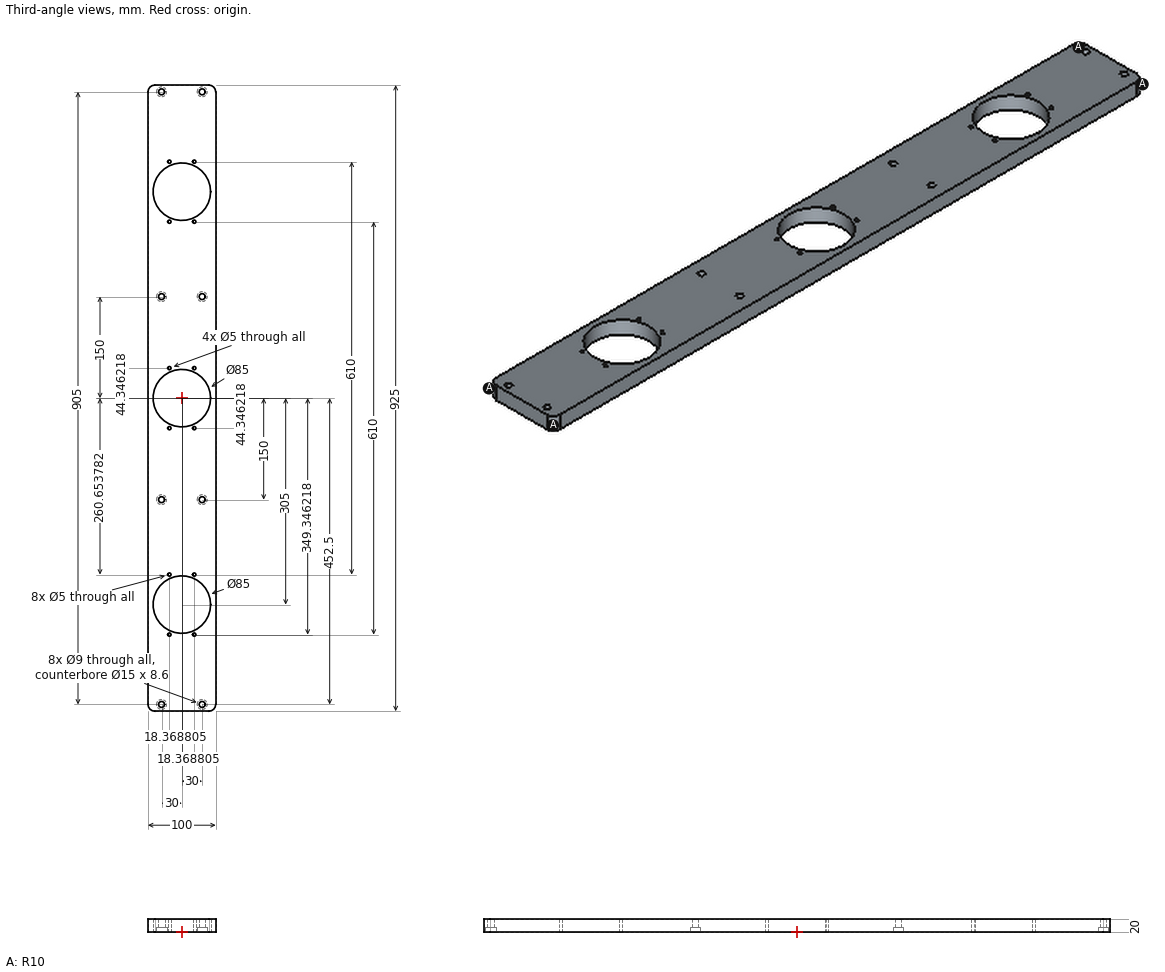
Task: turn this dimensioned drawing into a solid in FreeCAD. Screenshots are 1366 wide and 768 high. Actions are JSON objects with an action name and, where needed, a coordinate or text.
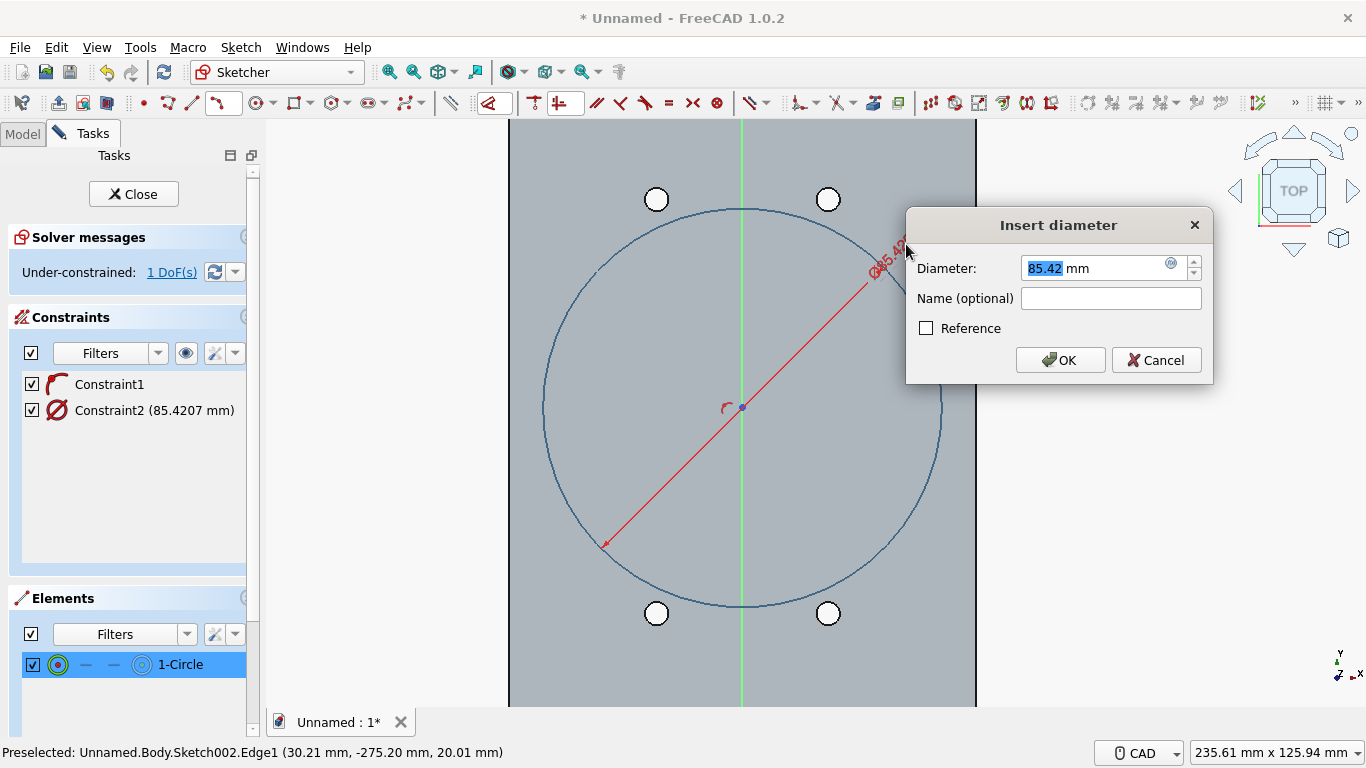
{"action": "type", "text": "85"}
{"action": "key", "text": "Return"}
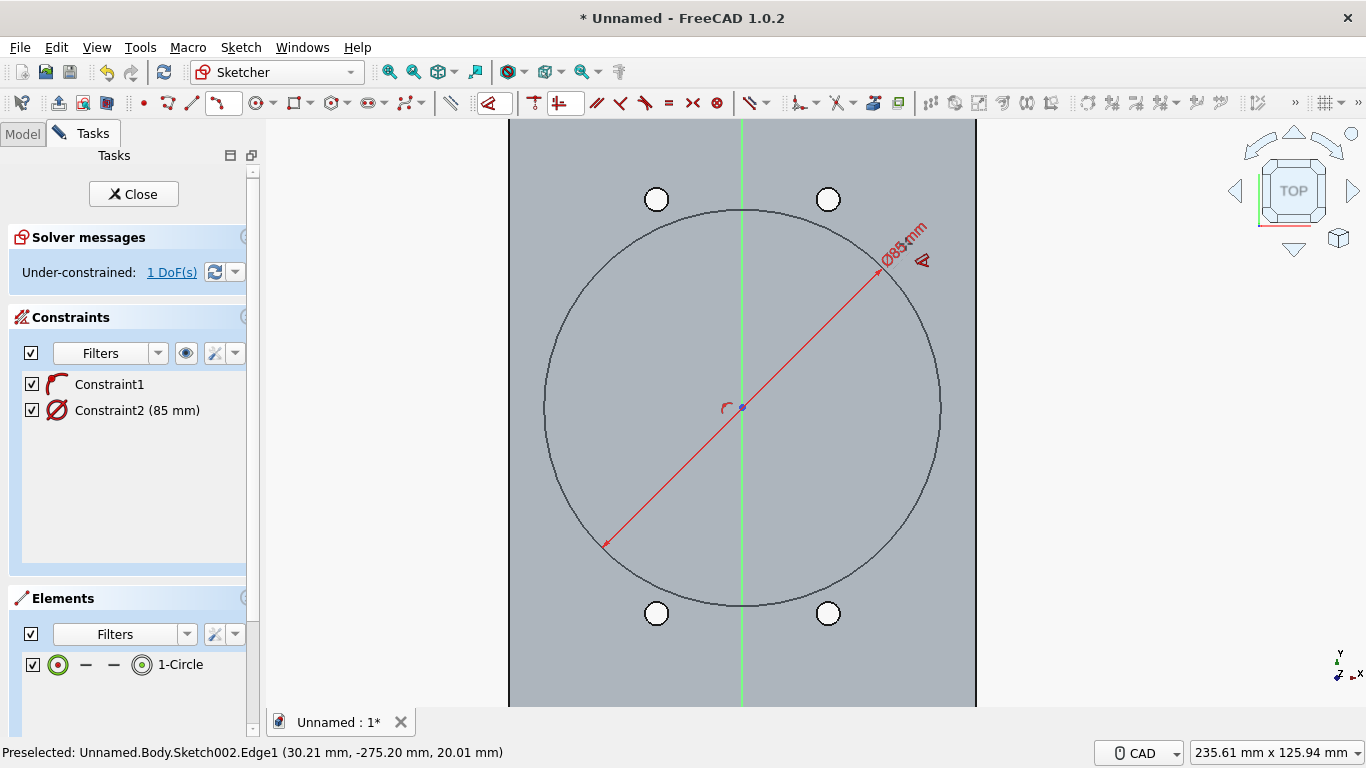
{"action": "left_click", "coordinate": [742, 408]}
{"action": "left_click", "coordinate": [776, 277]}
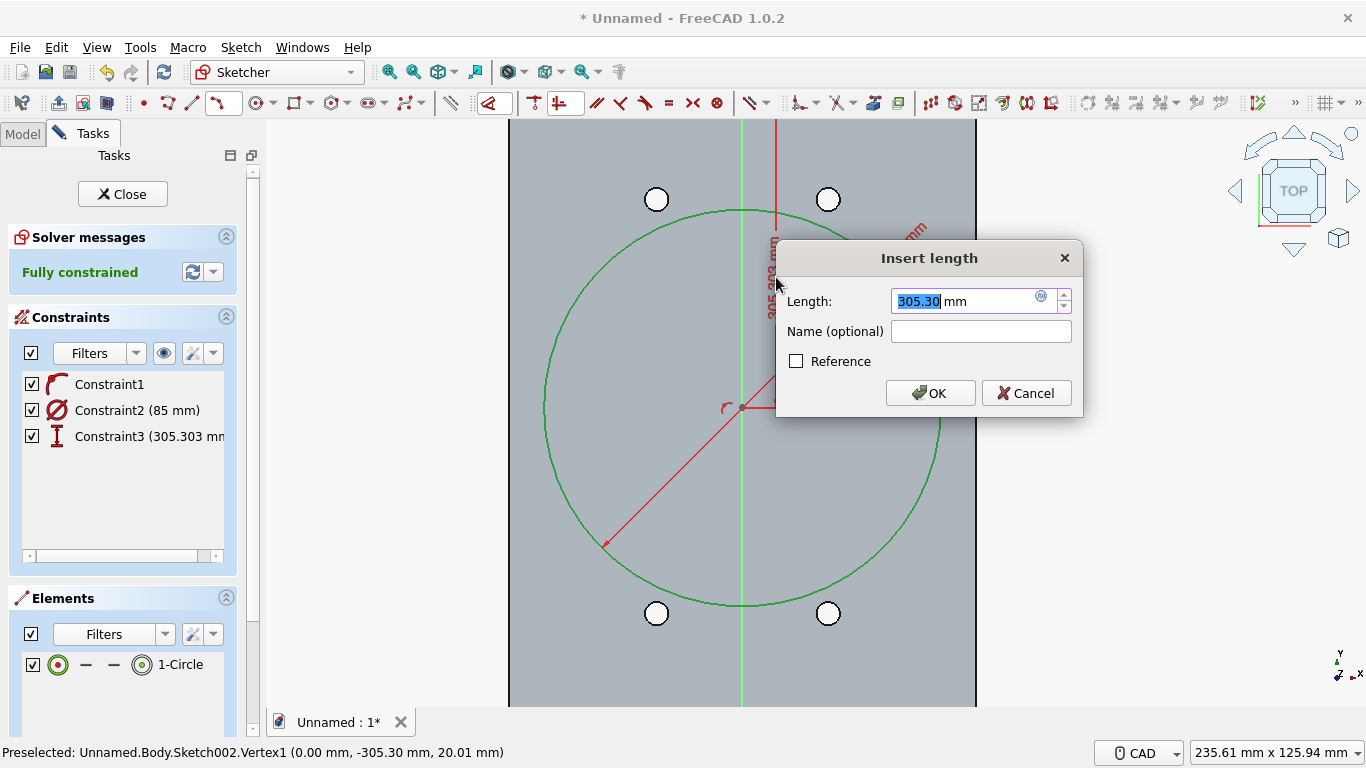
{"action": "type", "text": "305"}
{"action": "key", "text": "Return"}
{"action": "key", "text": "Escape"}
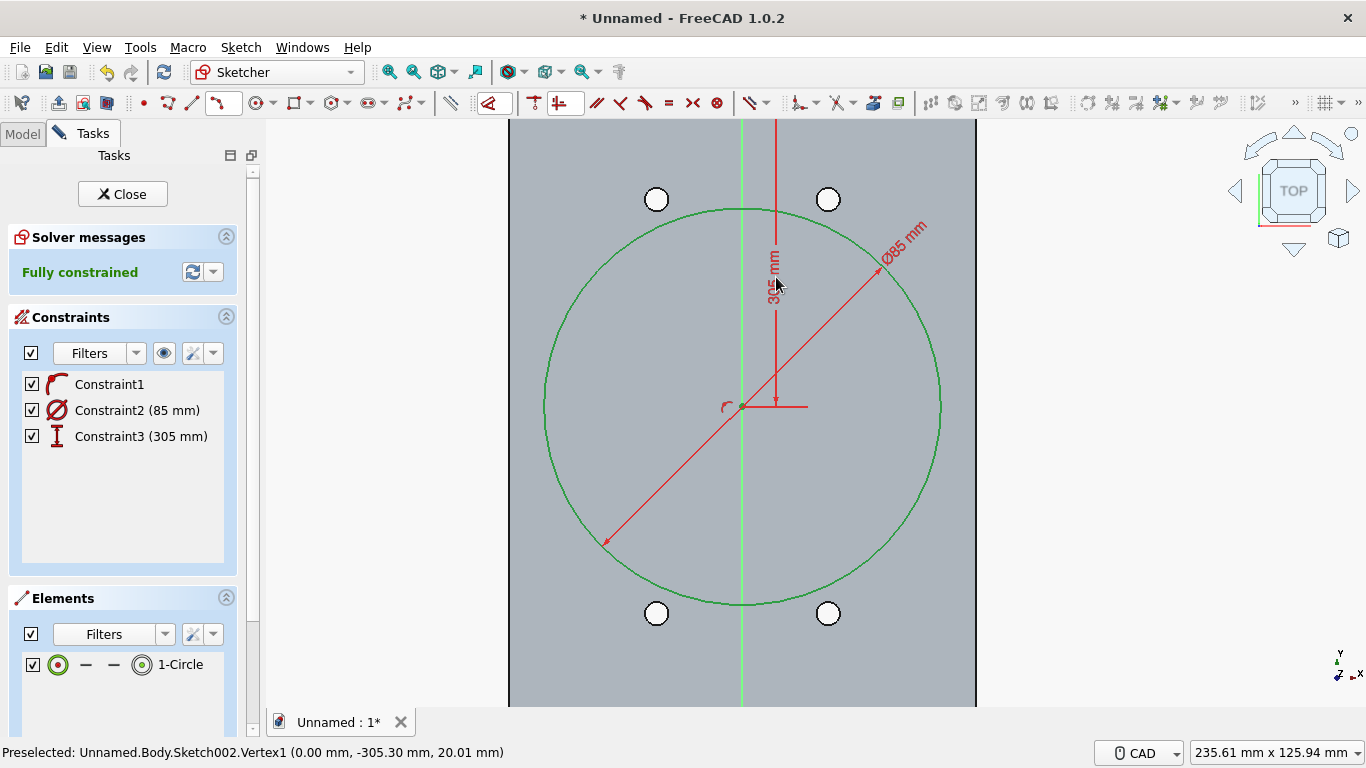
{"action": "left_click", "coordinate": [123, 194]}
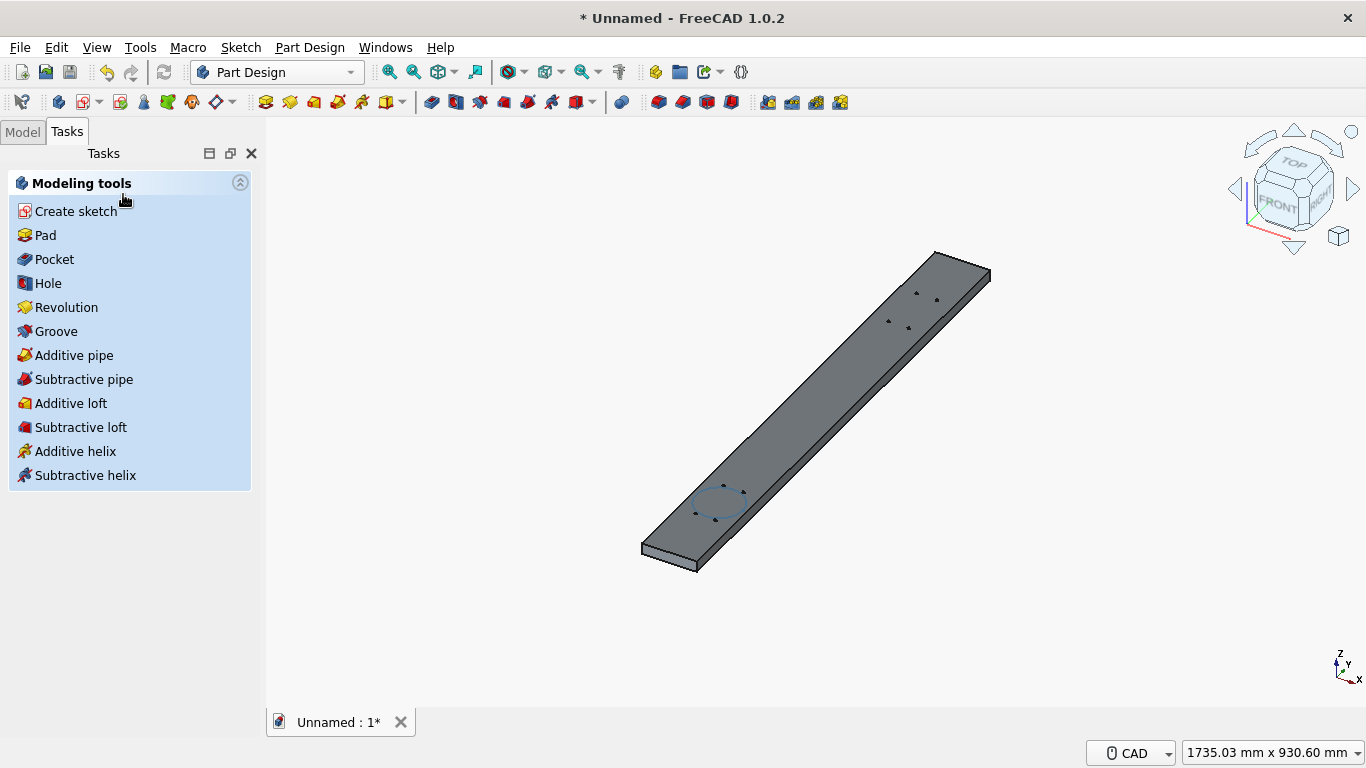
{"action": "left_click", "coordinate": [432, 102]}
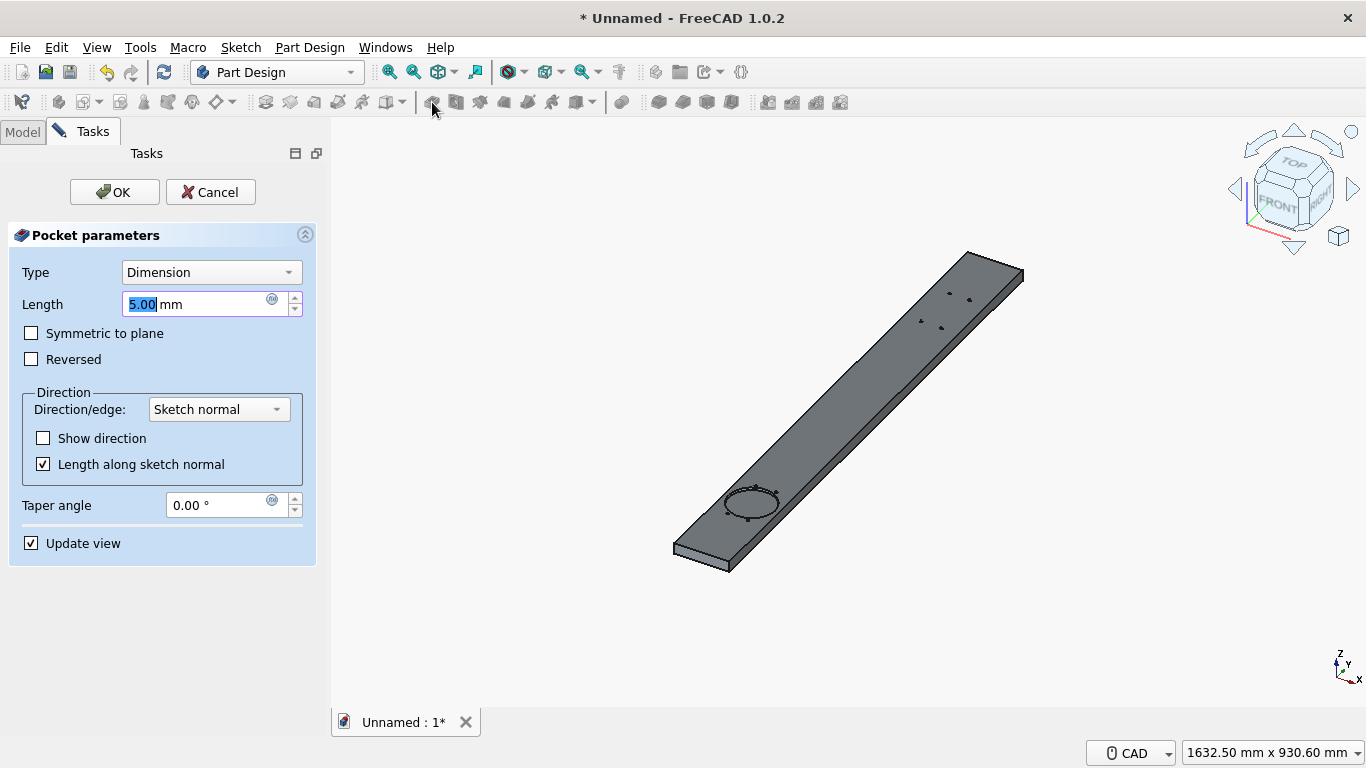
{"action": "left_click", "coordinate": [212, 272]}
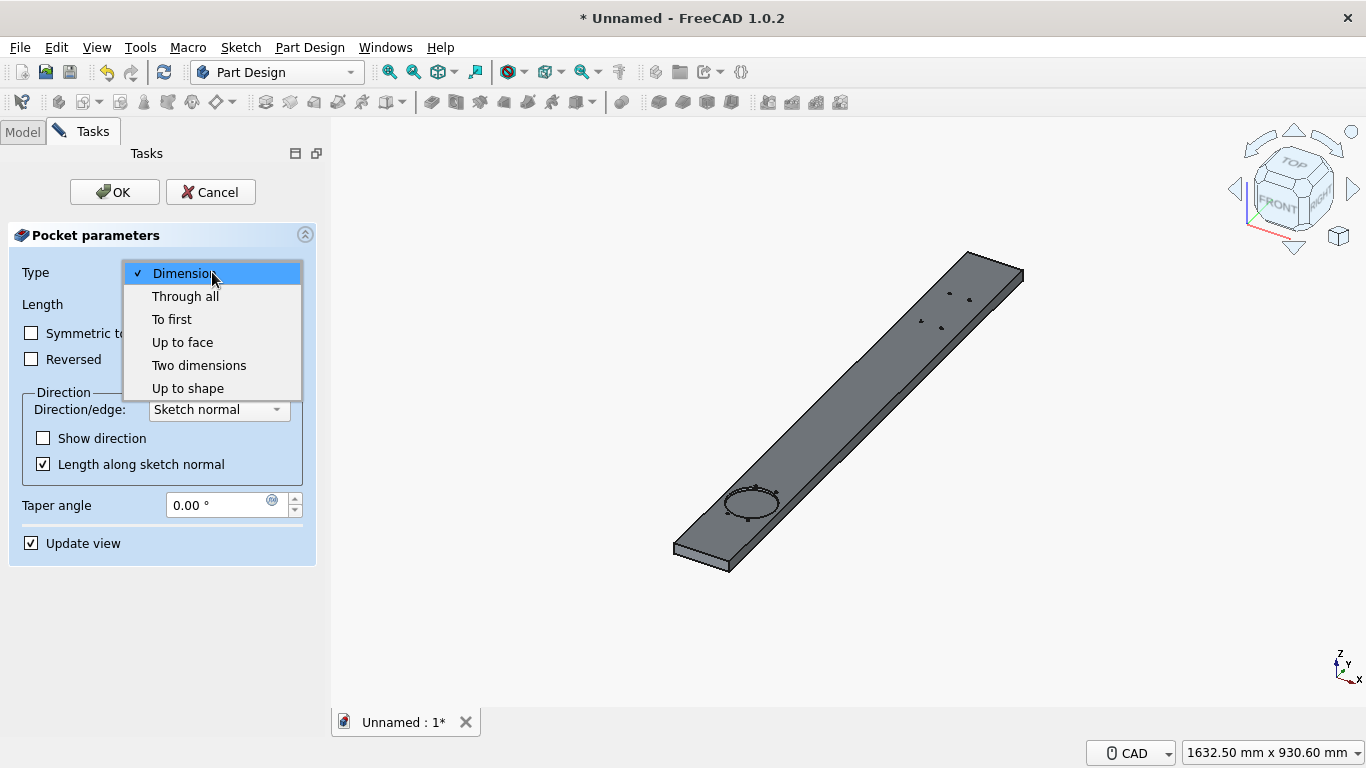
{"action": "left_click", "coordinate": [212, 296]}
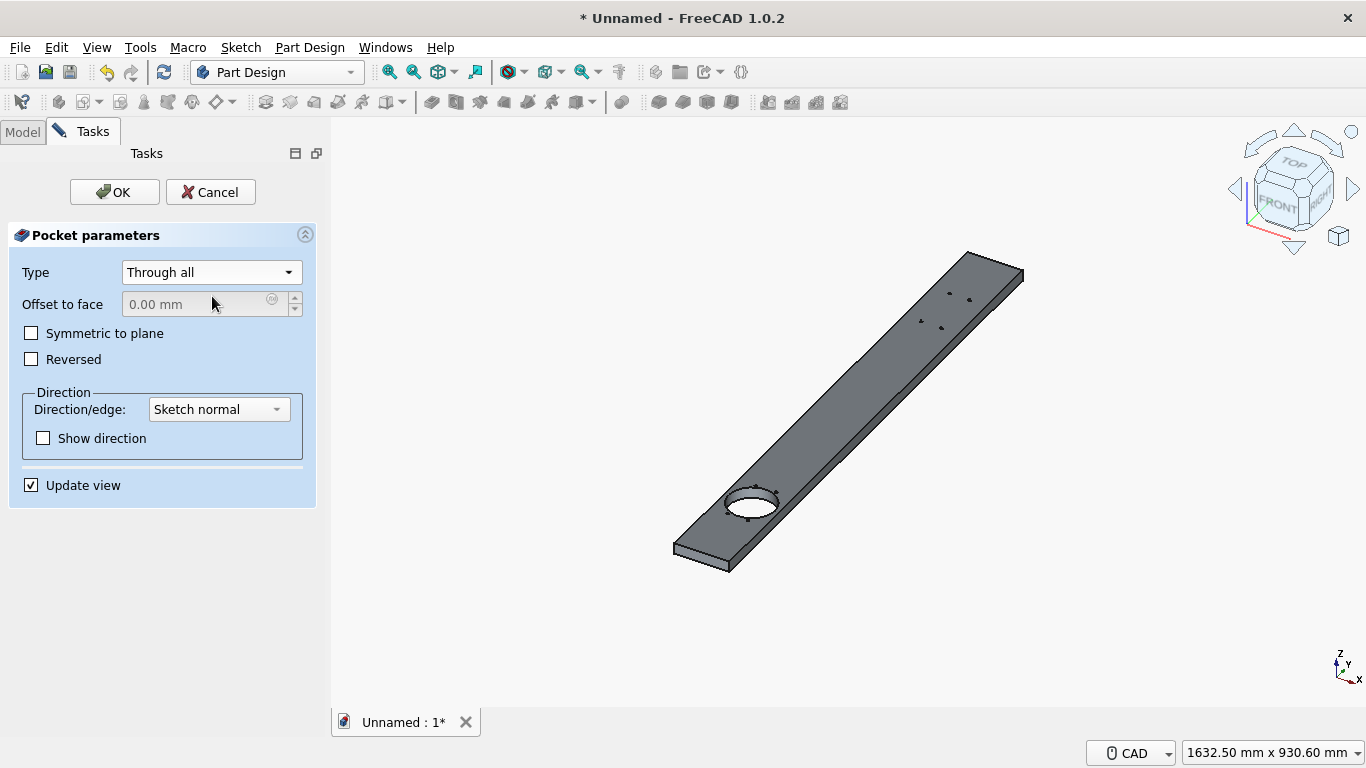
{"action": "left_click", "coordinate": [115, 192]}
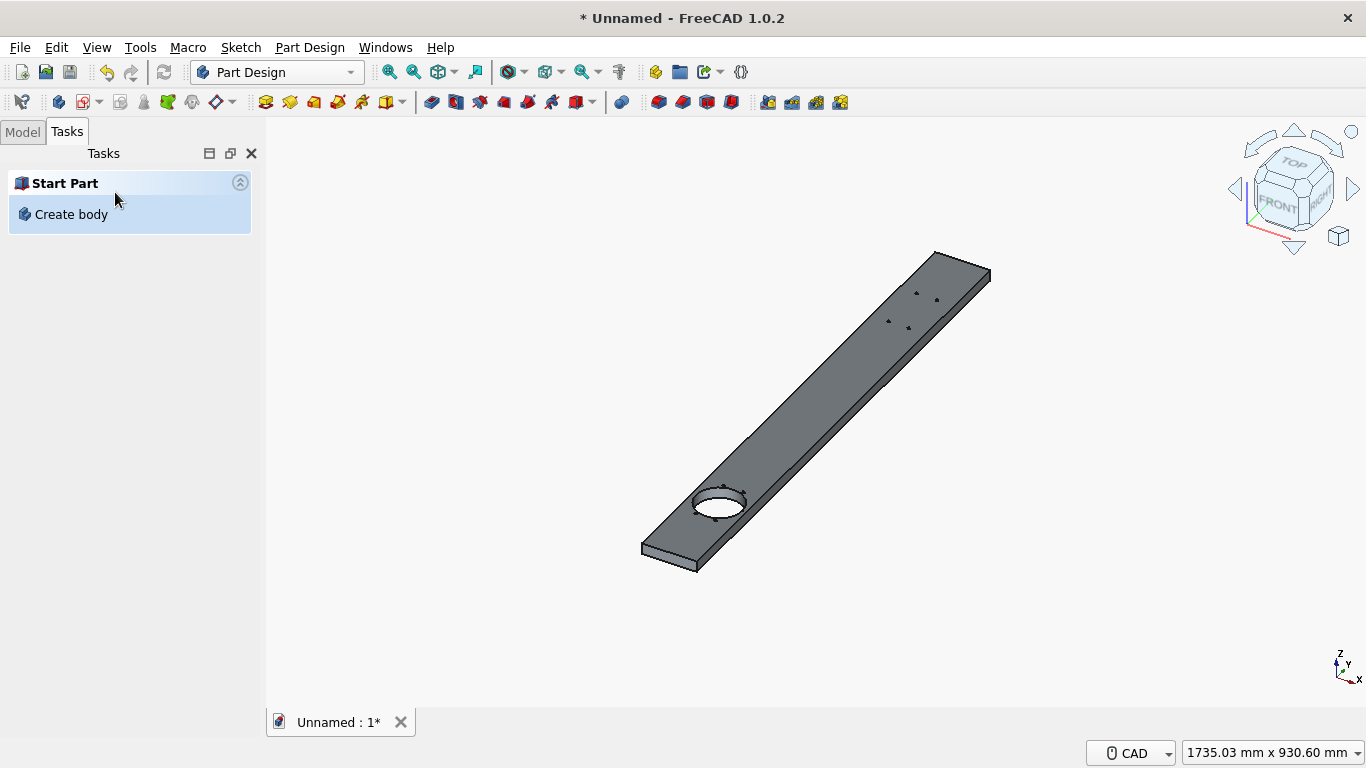
{"action": "key", "text": "5"}